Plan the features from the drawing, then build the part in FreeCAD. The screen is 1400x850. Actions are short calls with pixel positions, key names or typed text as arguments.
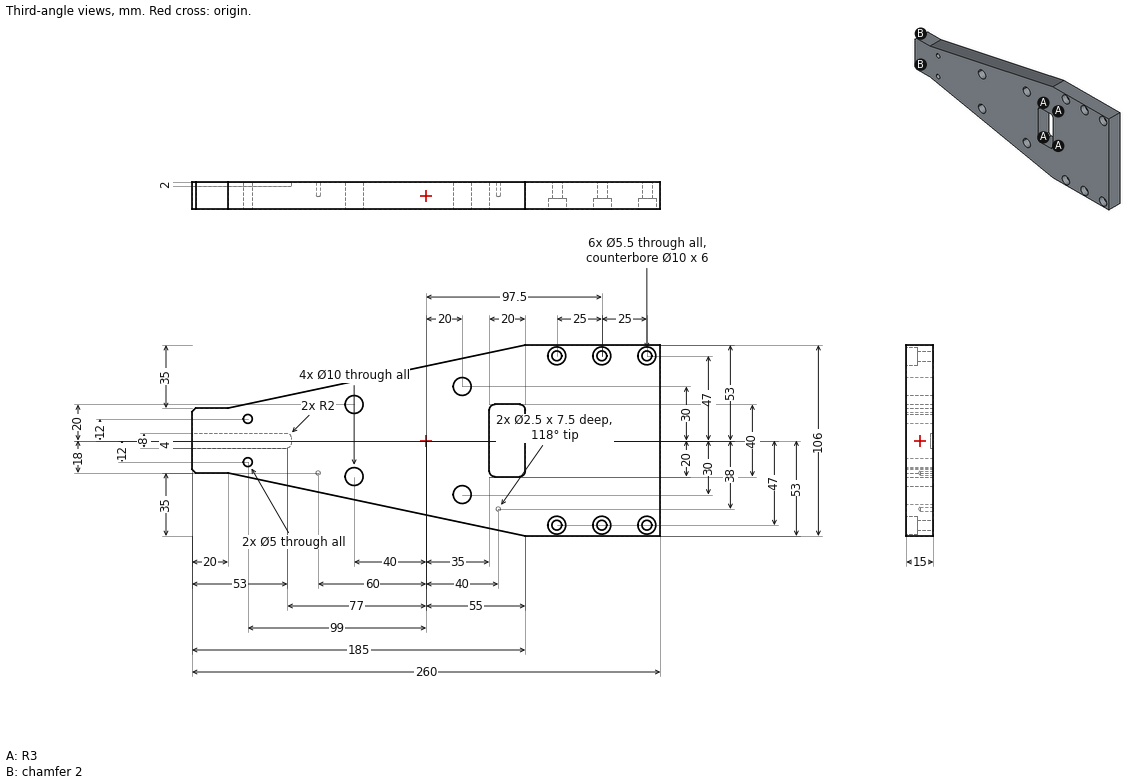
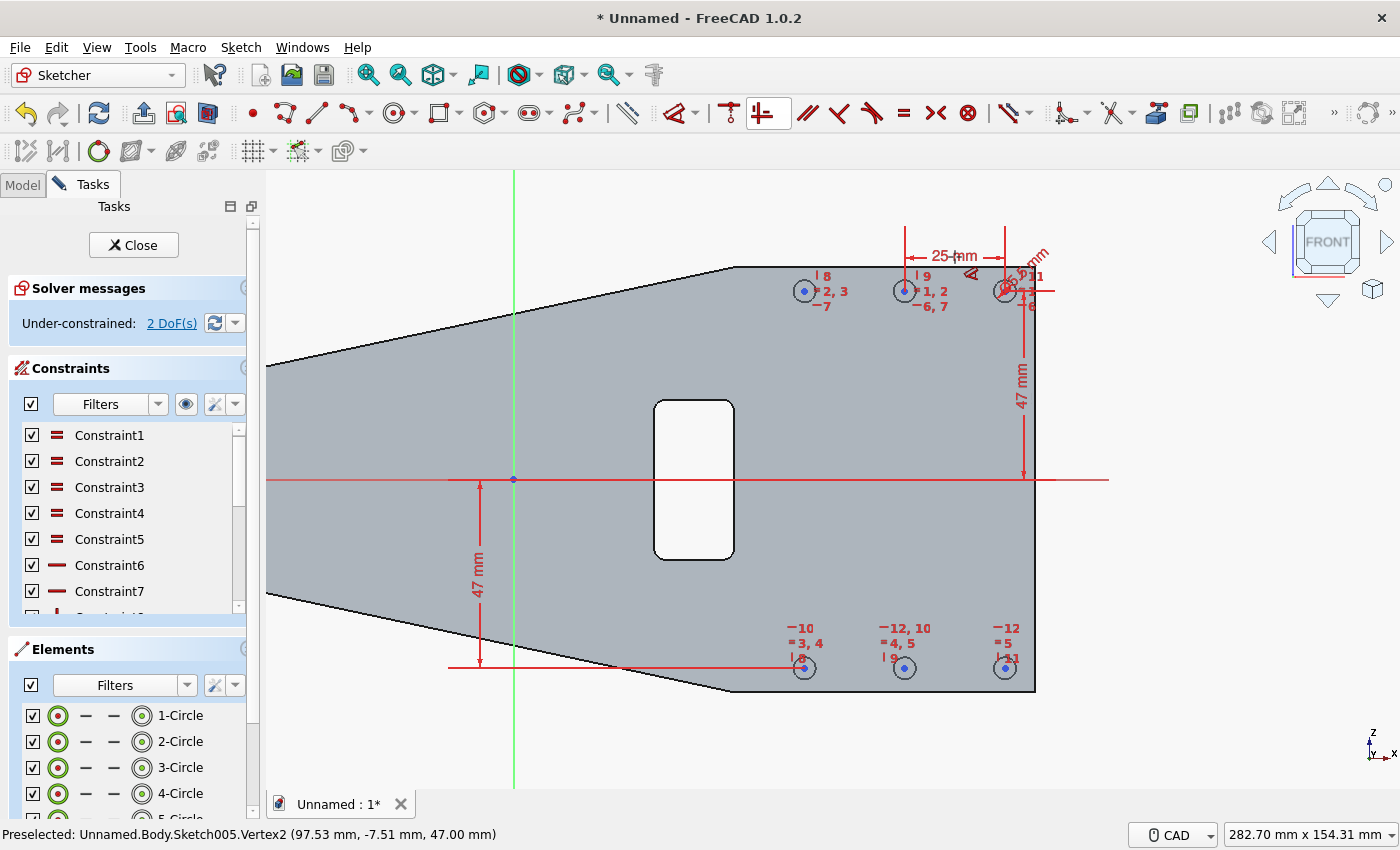
click(905, 291)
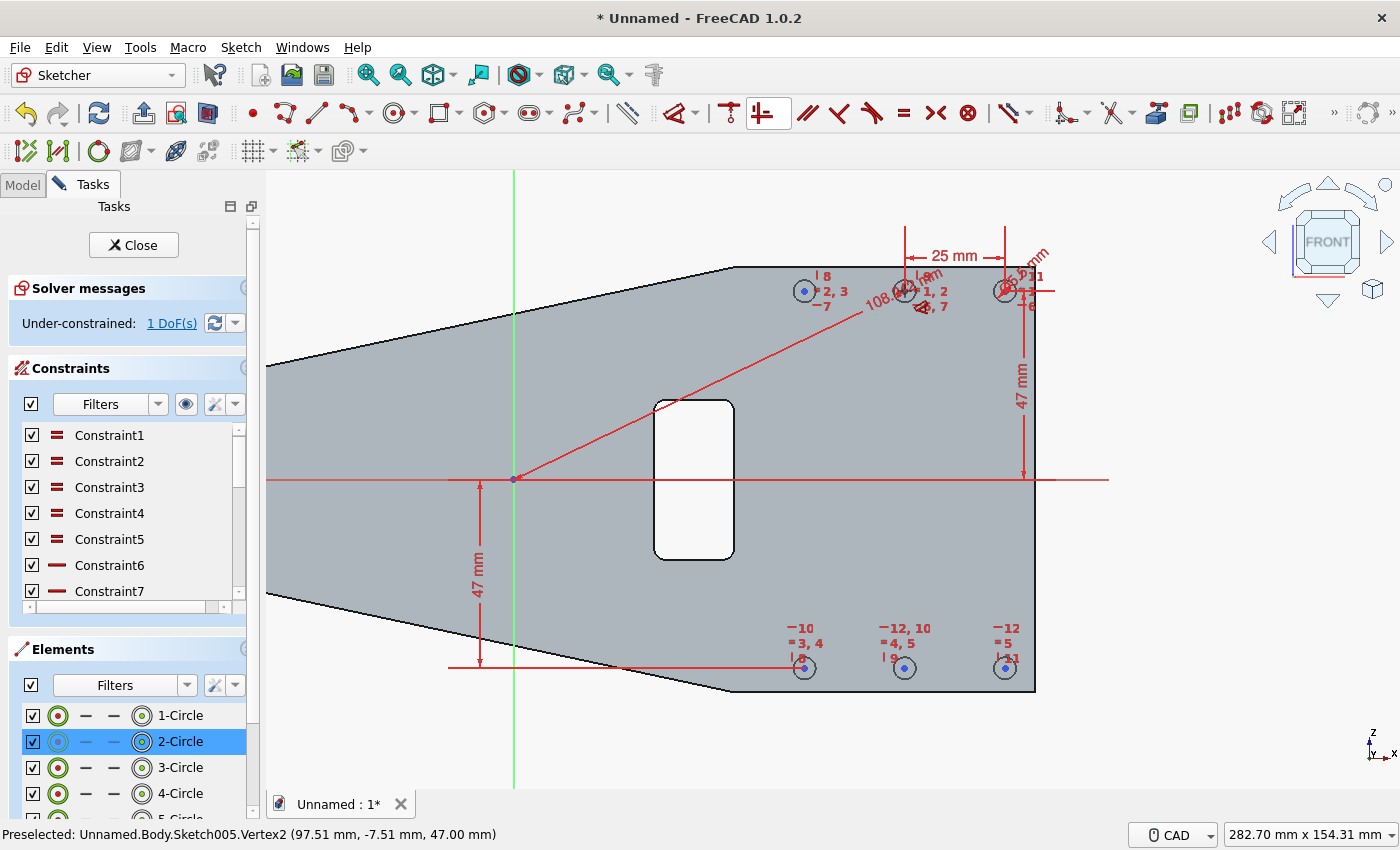
click(805, 291)
click(855, 257)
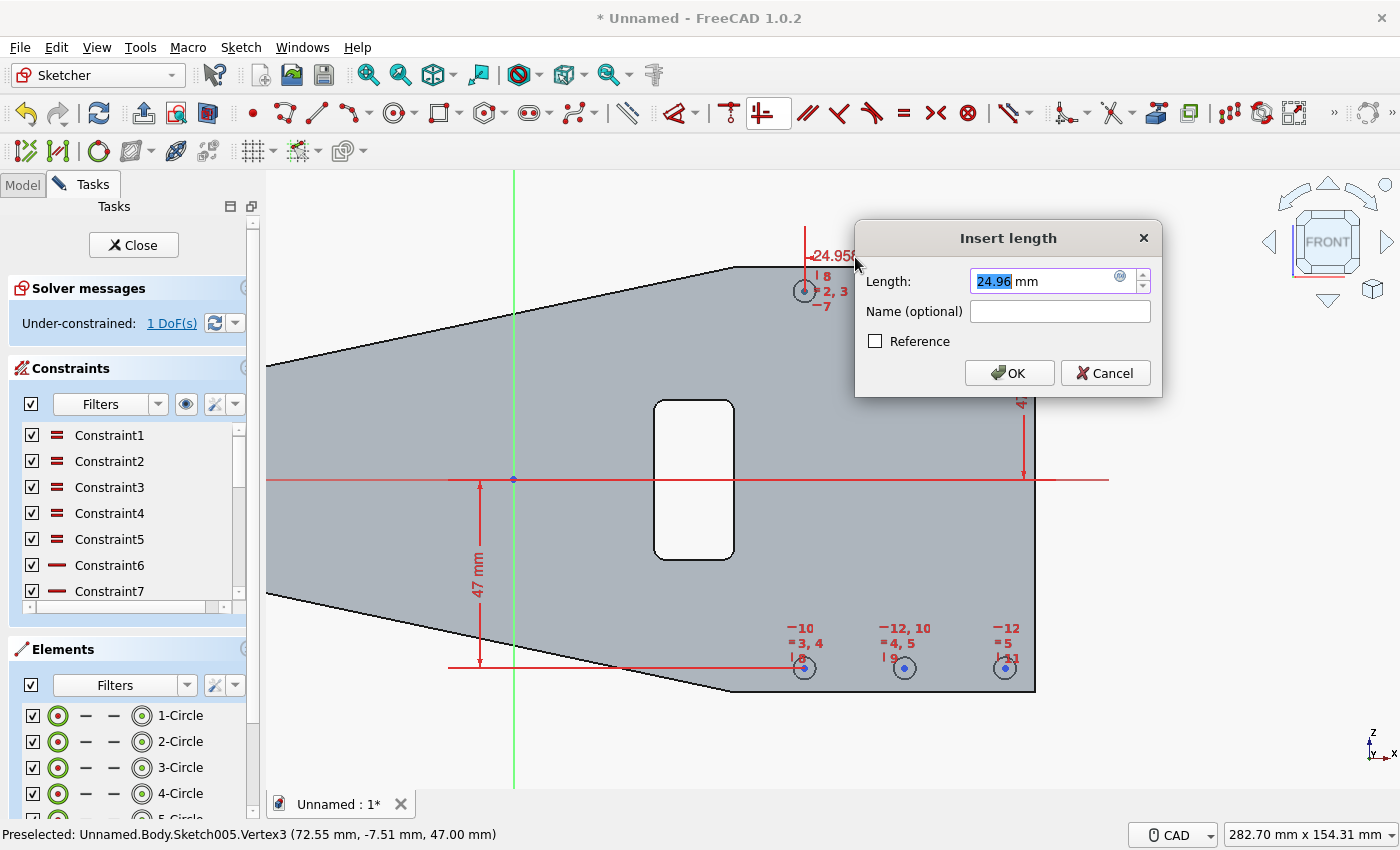
text(25)
key(Return)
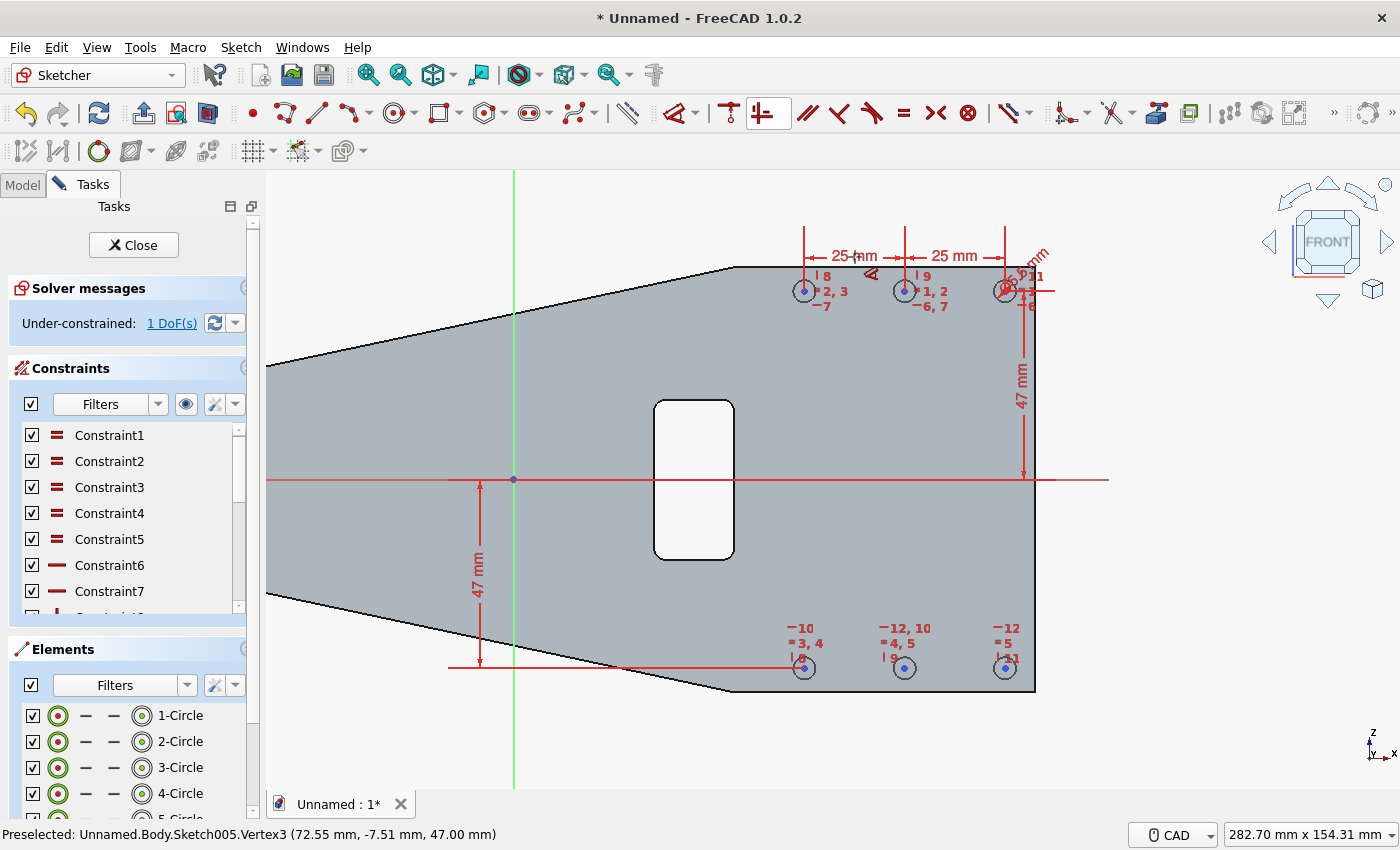
click(905, 291)
click(709, 257)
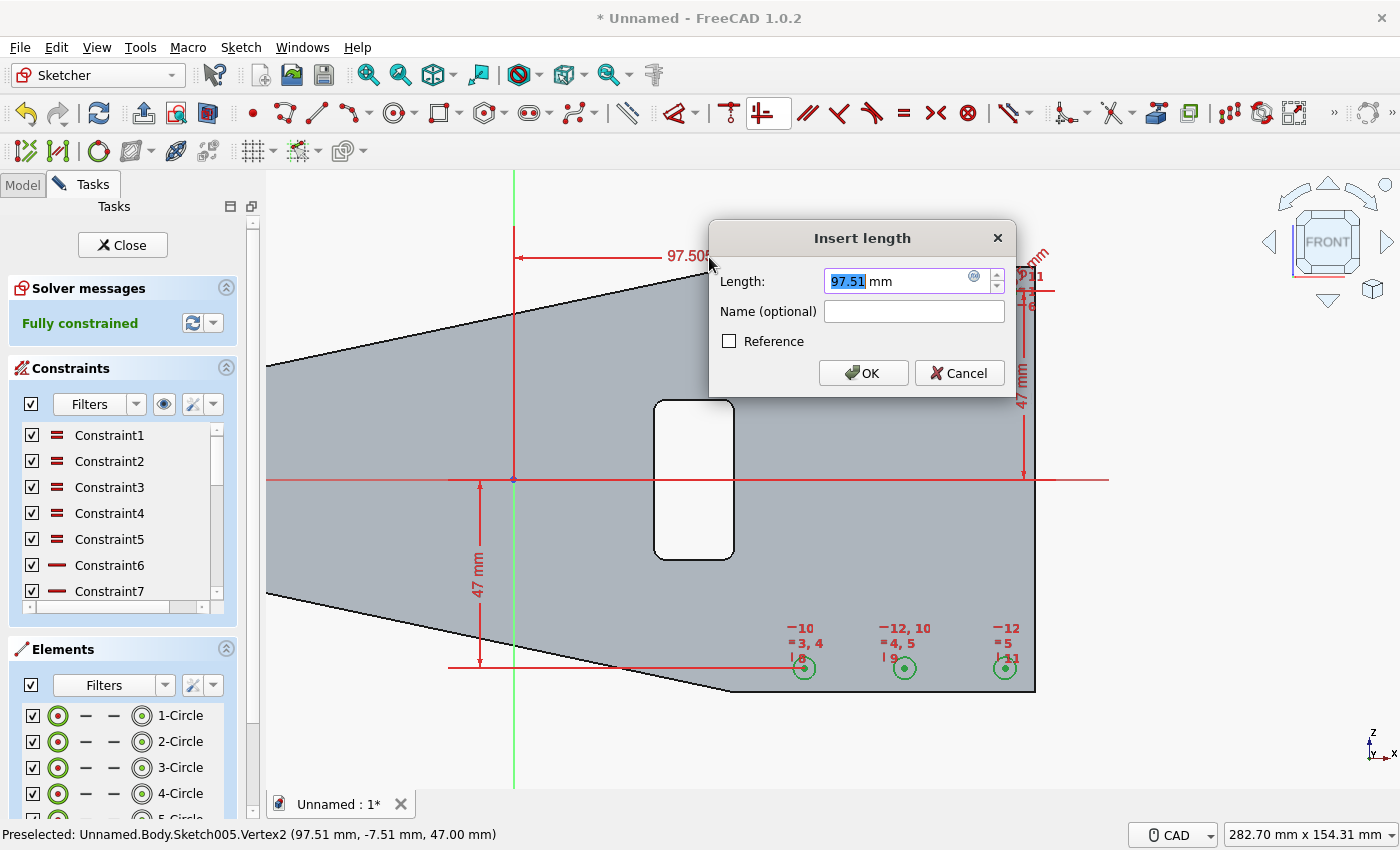
text(97.5)
key(Return)
key(Escape)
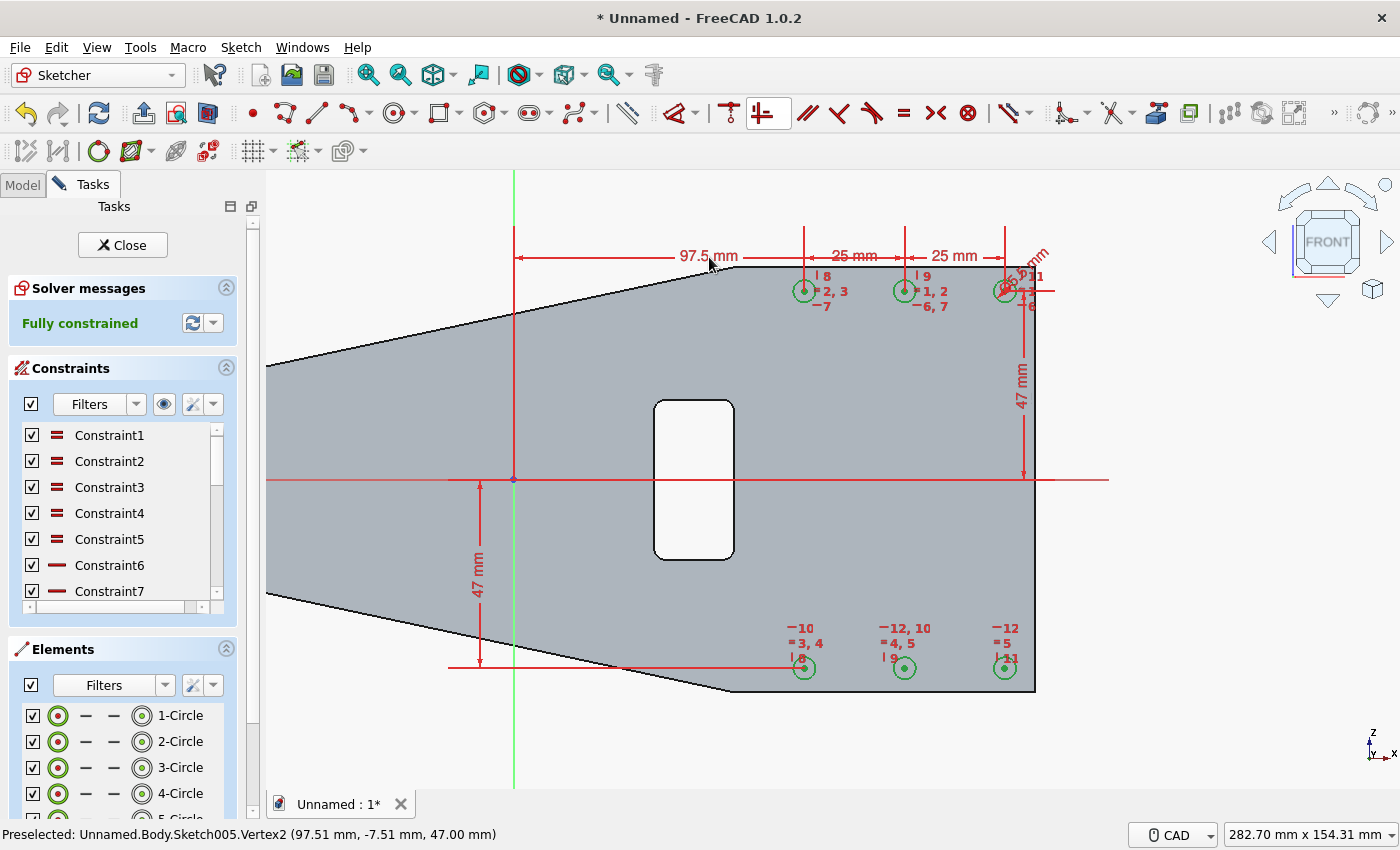
click(123, 245)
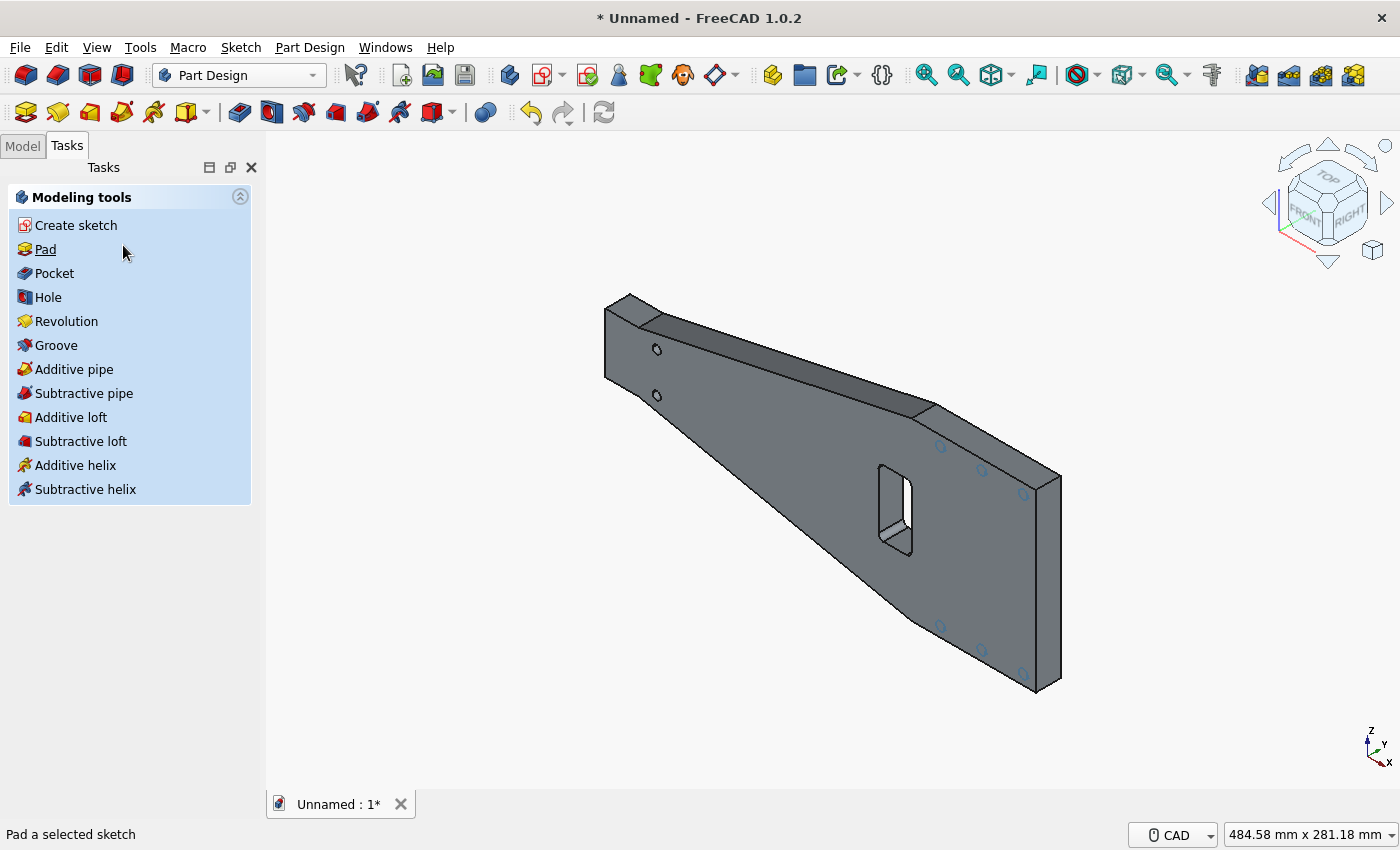
click(272, 112)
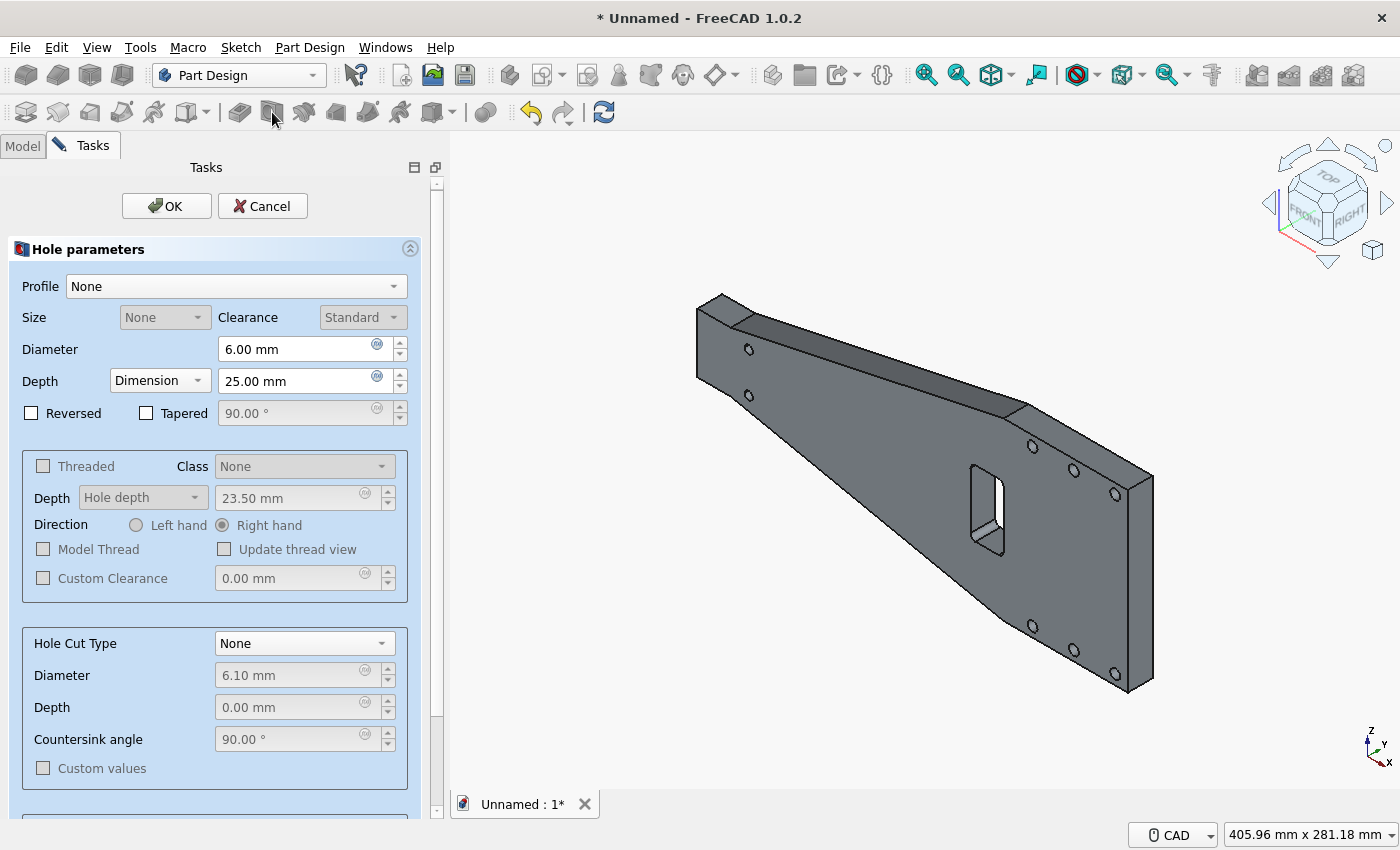
triple_click(305, 349)